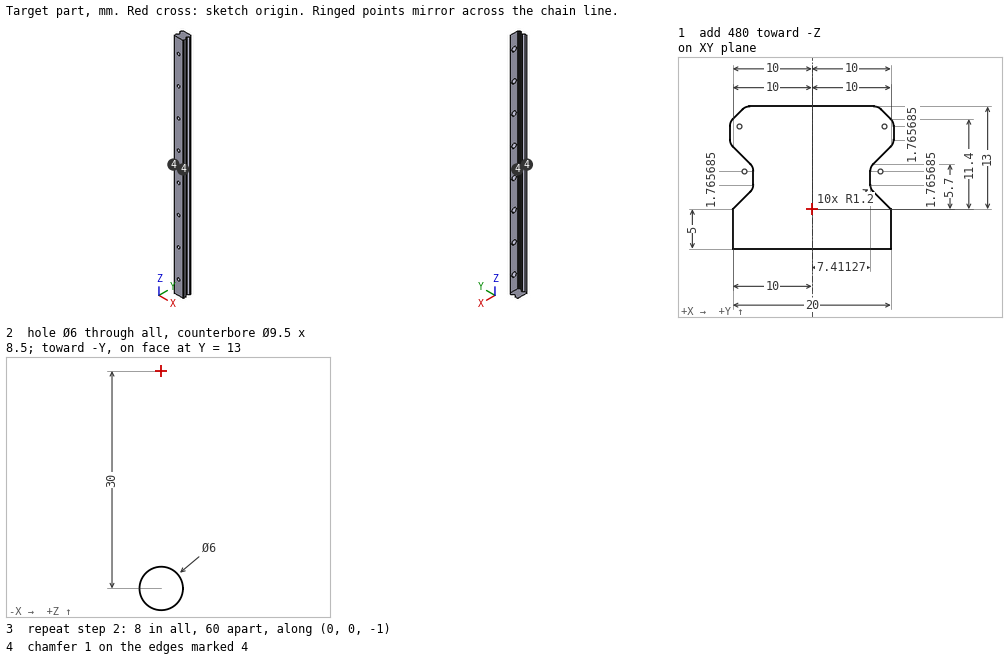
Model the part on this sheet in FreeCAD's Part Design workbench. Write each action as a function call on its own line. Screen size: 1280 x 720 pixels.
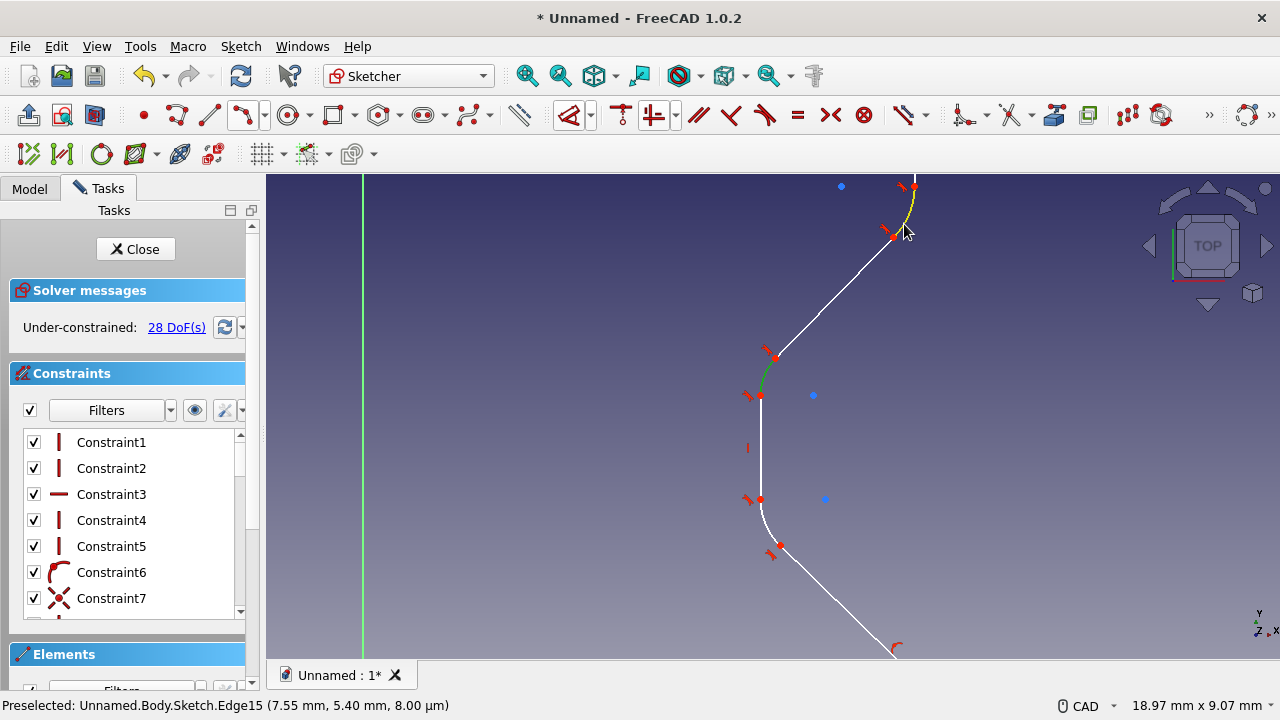
click(904, 224)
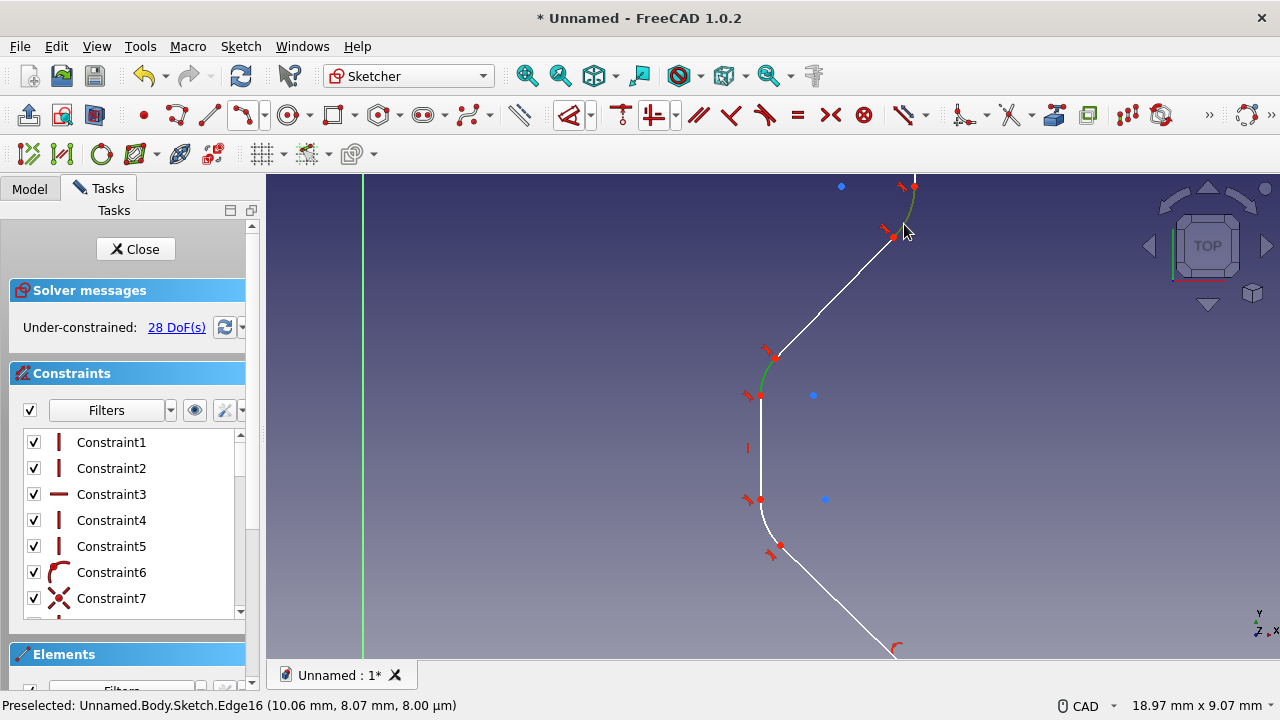
scroll(852, 404, down, 6)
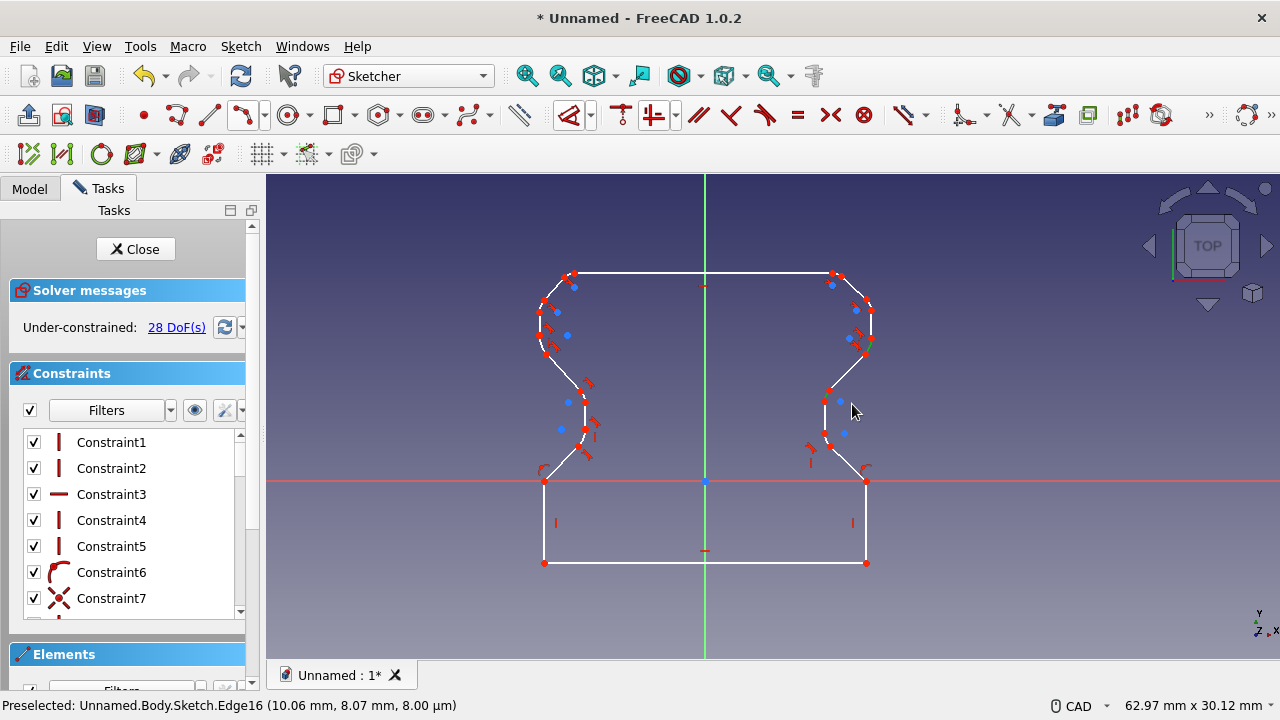
scroll(871, 307, up, 7)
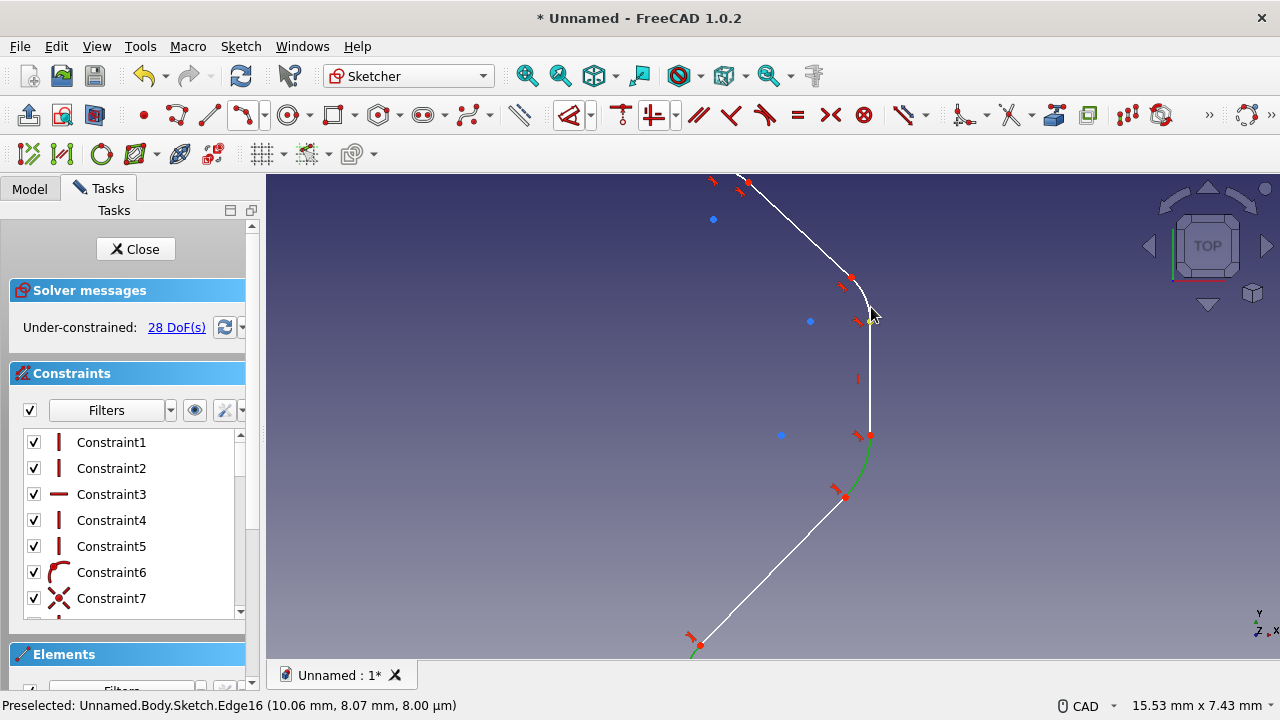
click(868, 307)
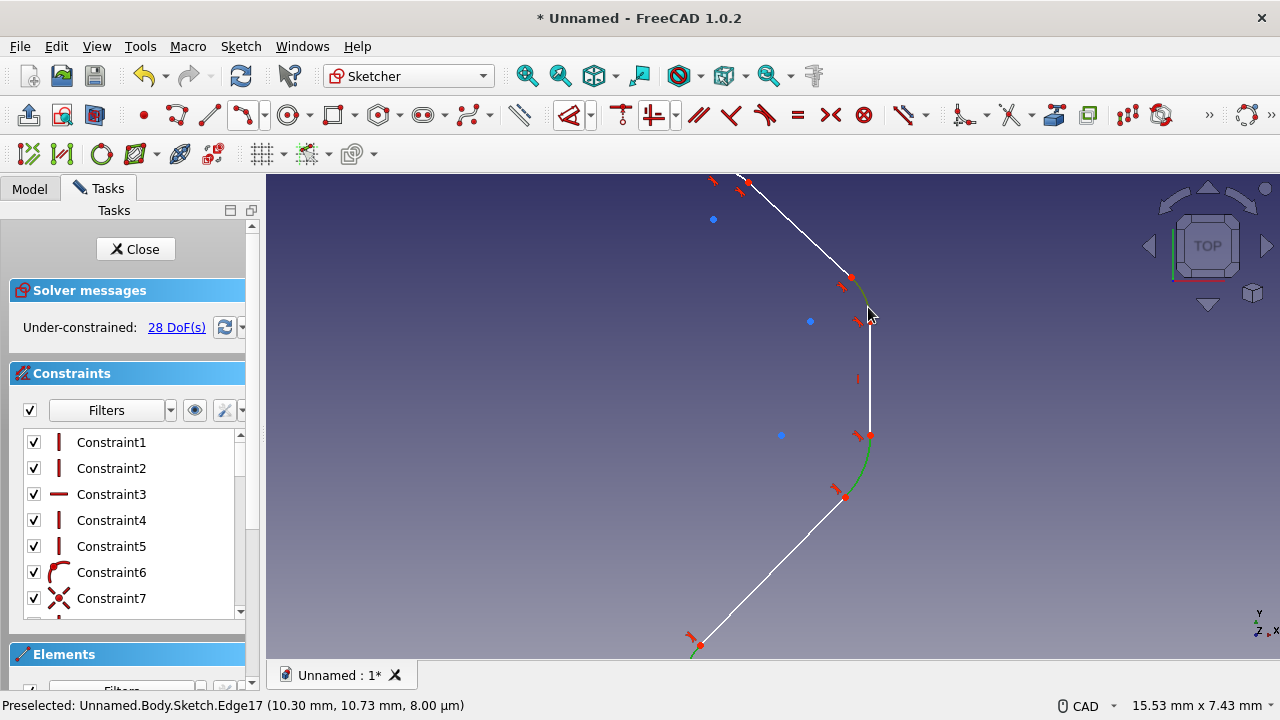
scroll(871, 307, down, 7)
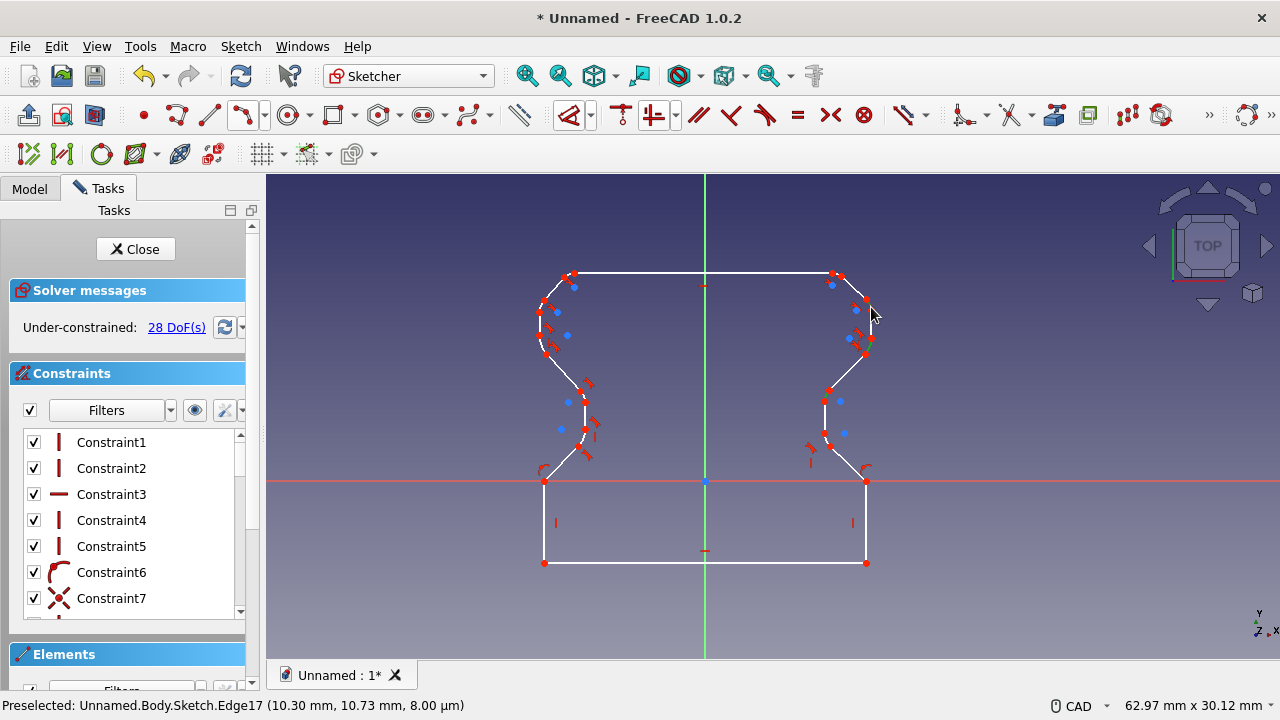
scroll(839, 275, up, 8)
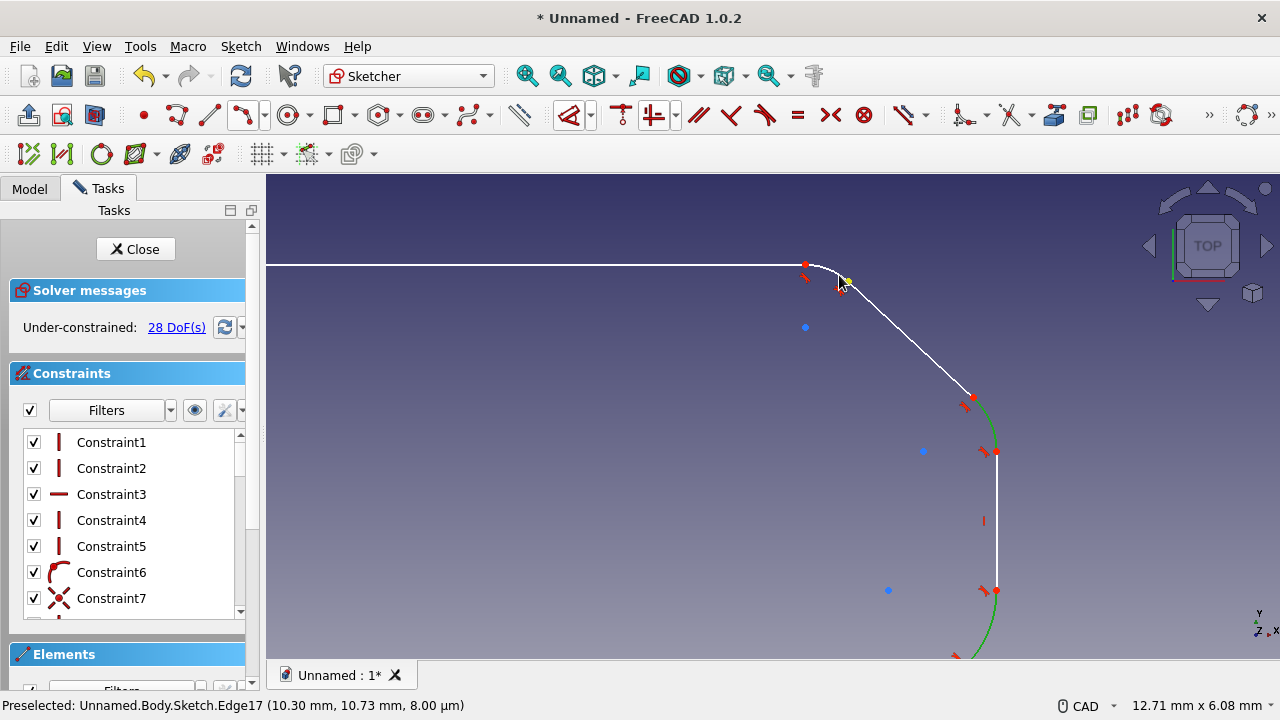
click(837, 273)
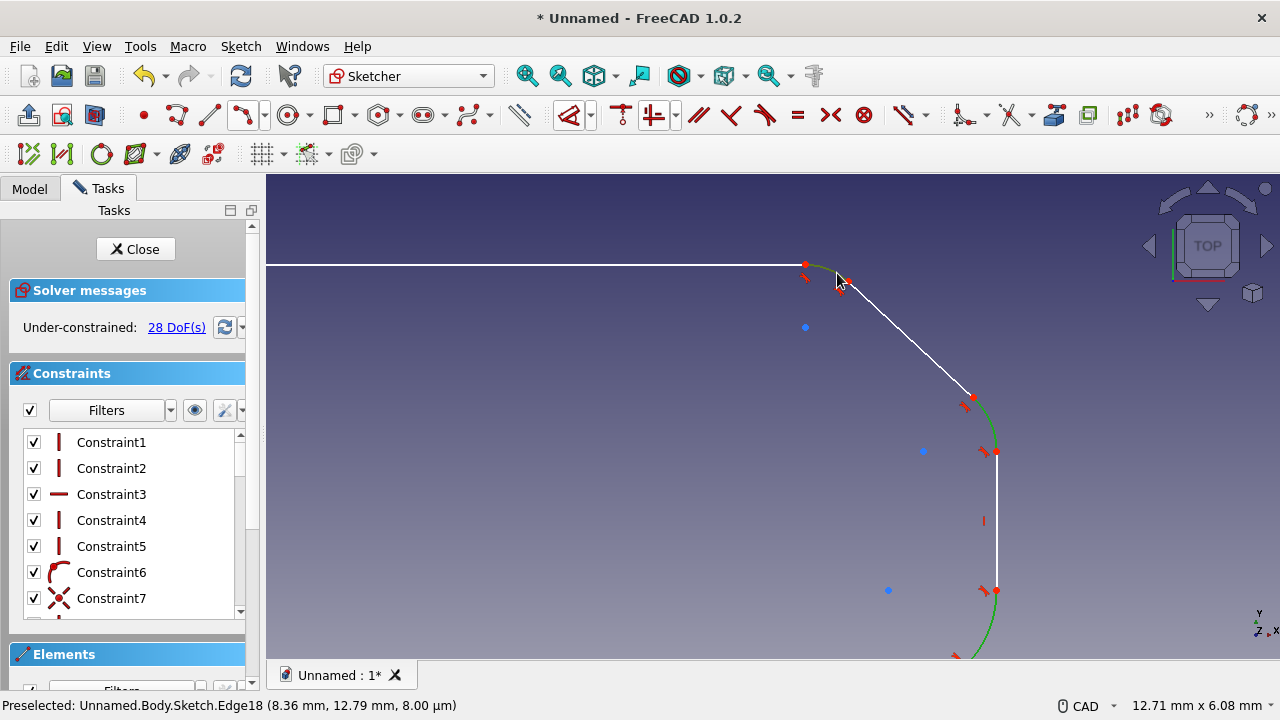
scroll(839, 275, down, 8)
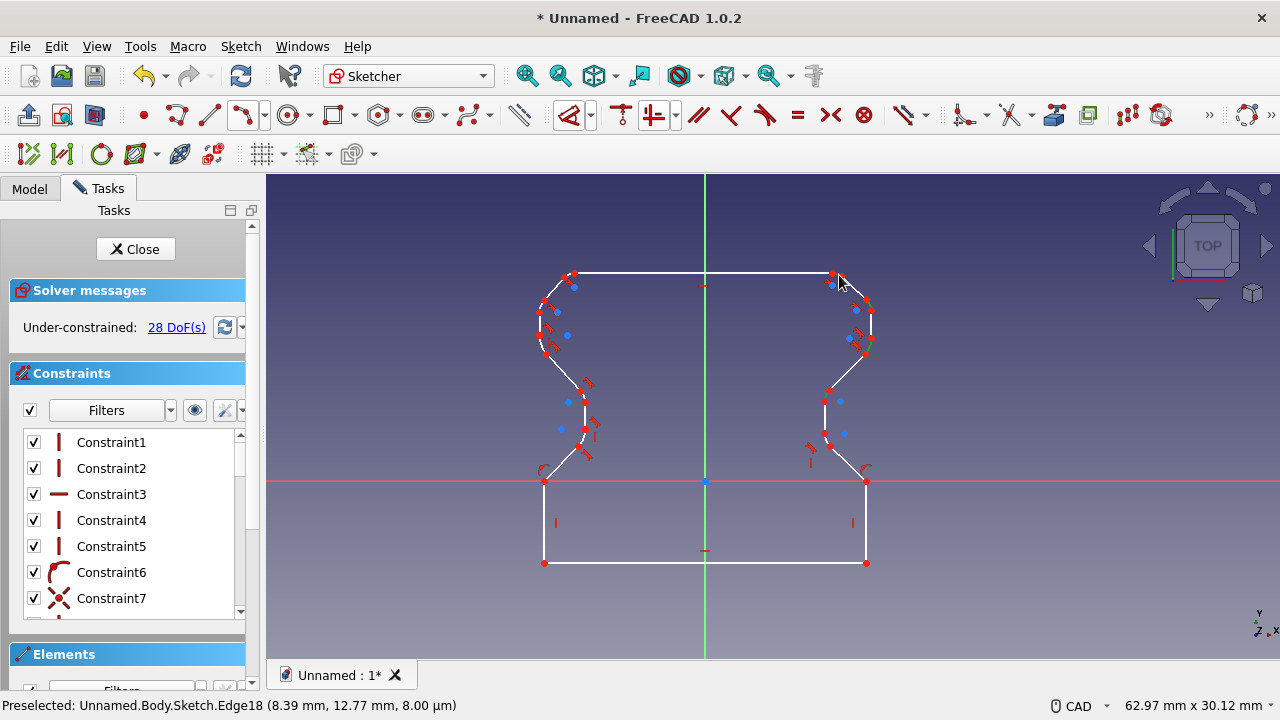
scroll(571, 274, up, 7)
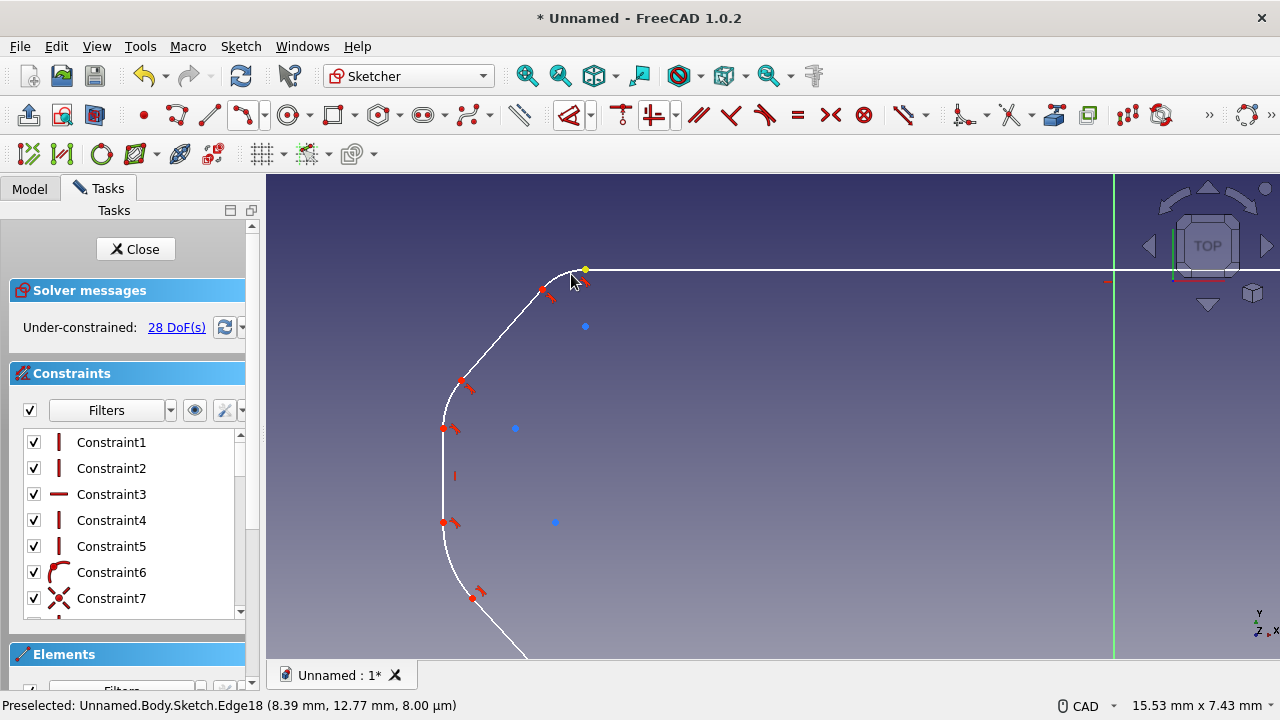
click(571, 272)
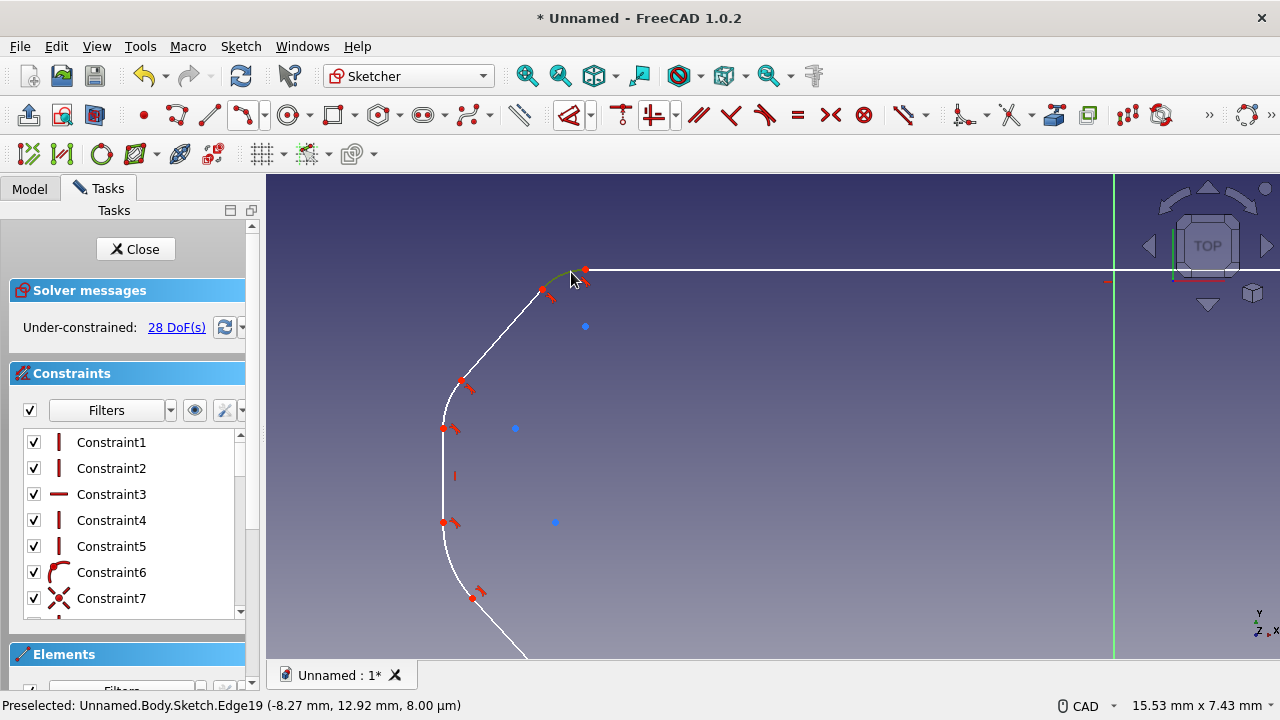
click(452, 394)